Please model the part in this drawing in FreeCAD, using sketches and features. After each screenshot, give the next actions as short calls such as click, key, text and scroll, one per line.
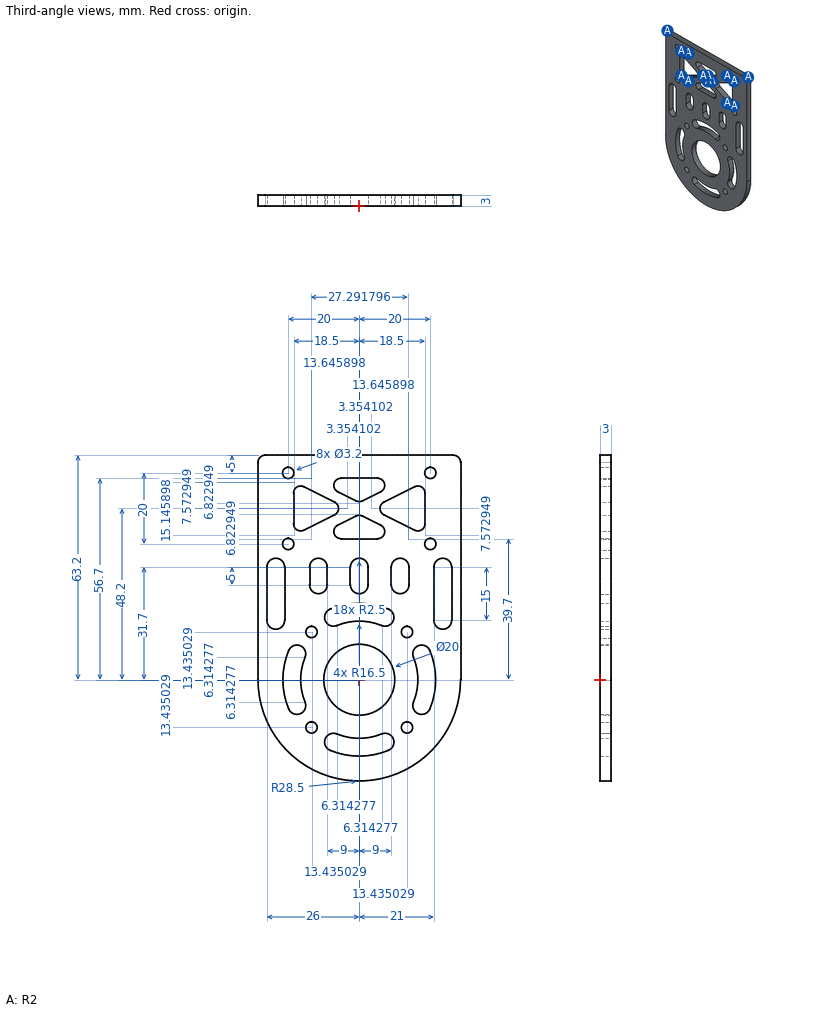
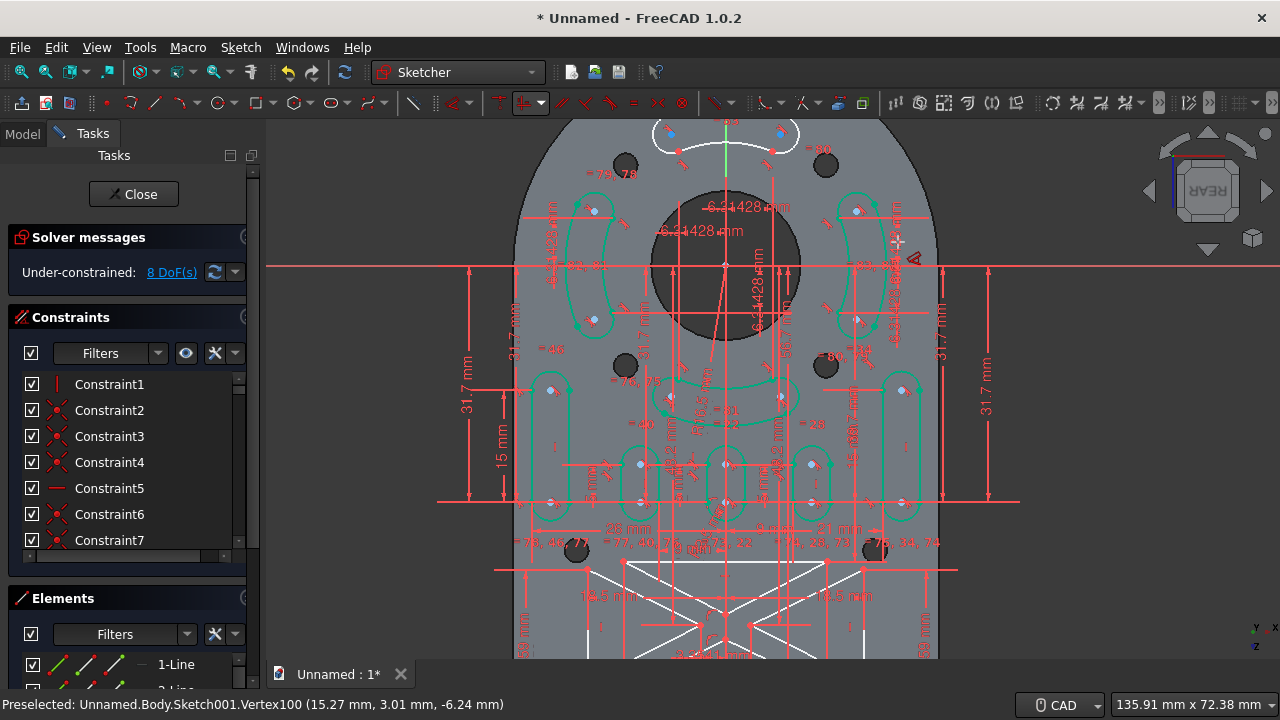
click(773, 152)
click(749, 372)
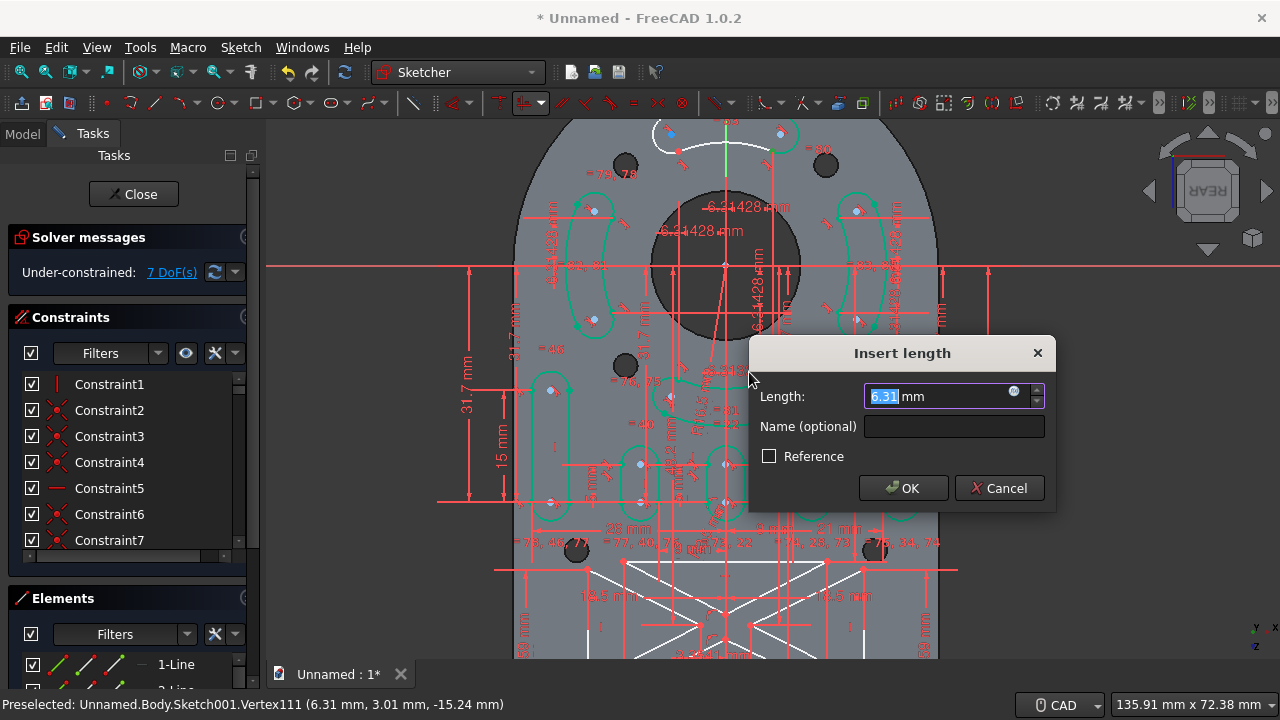
text(6.314277)
key(Return)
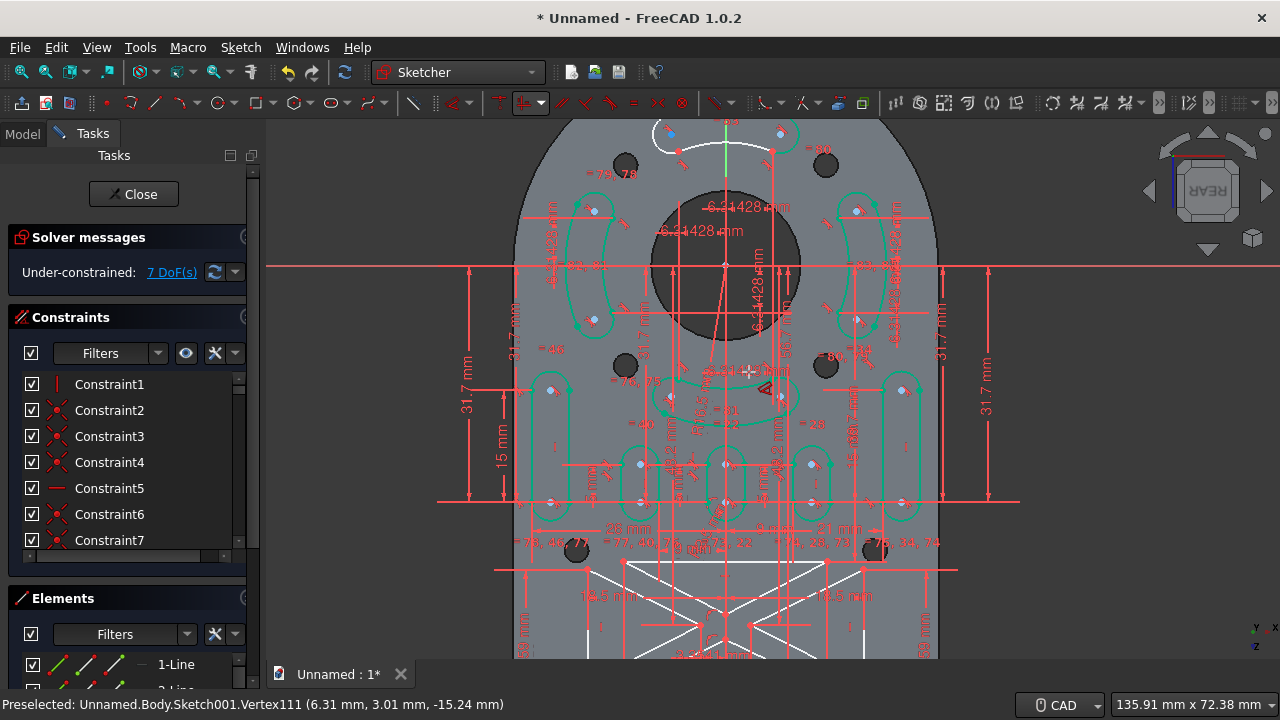
click(679, 152)
click(686, 300)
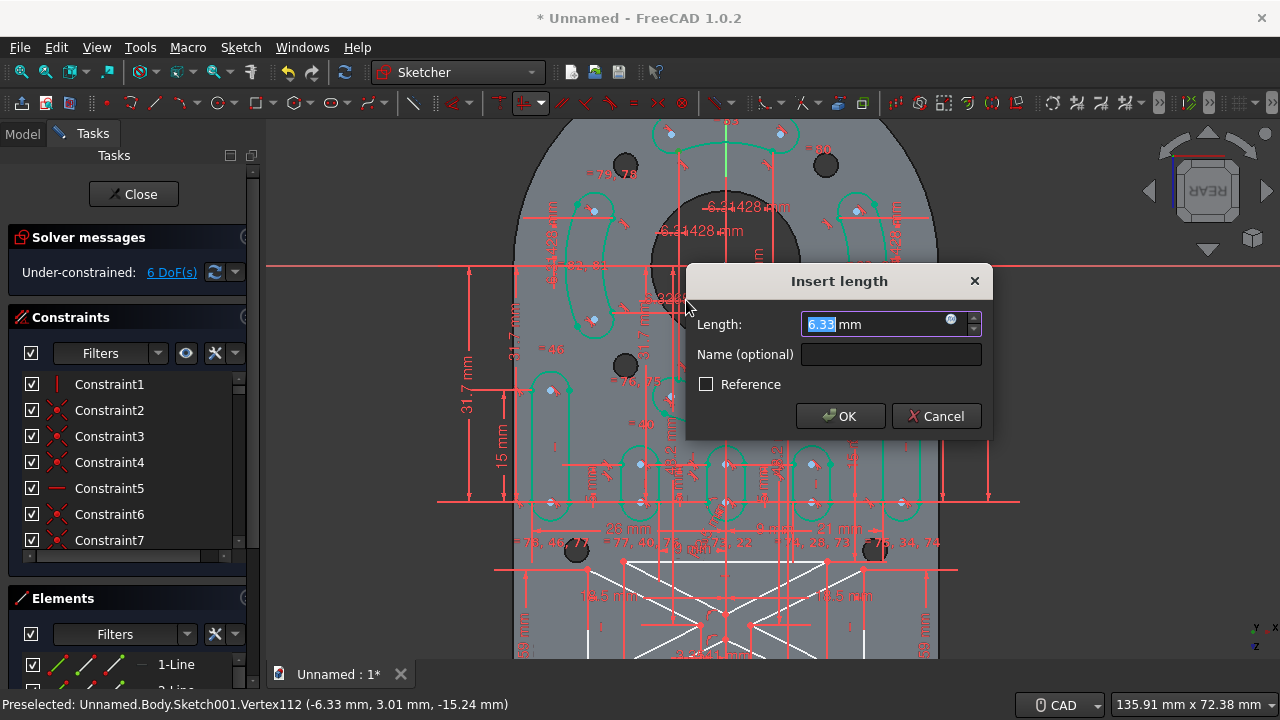
text(6.314277)
key(Return)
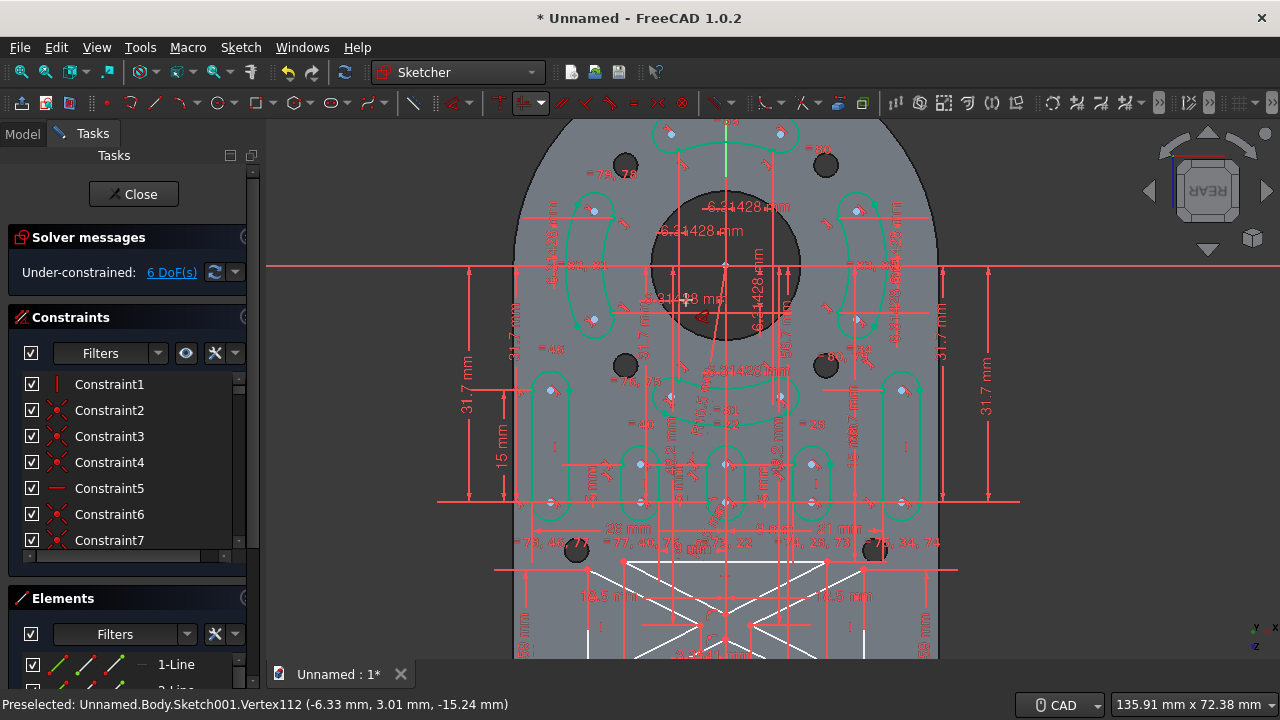
scroll(678, 379, down, 3)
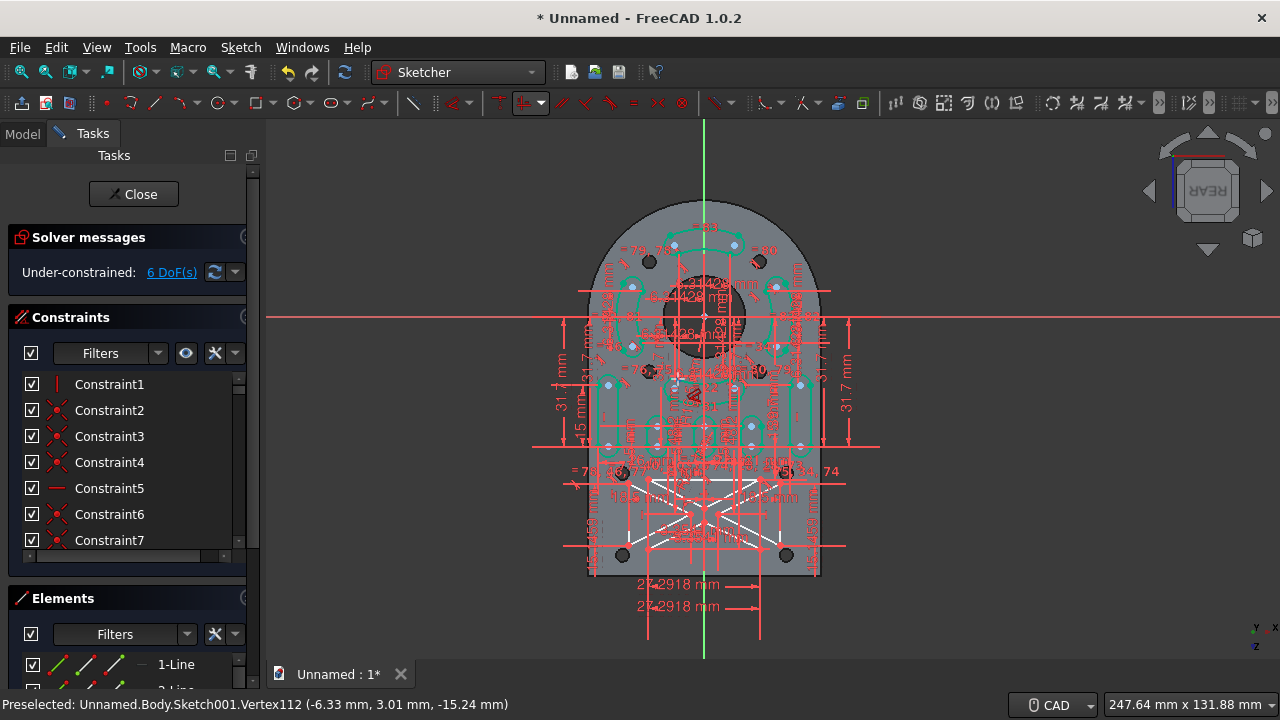
scroll(647, 536, up, 2)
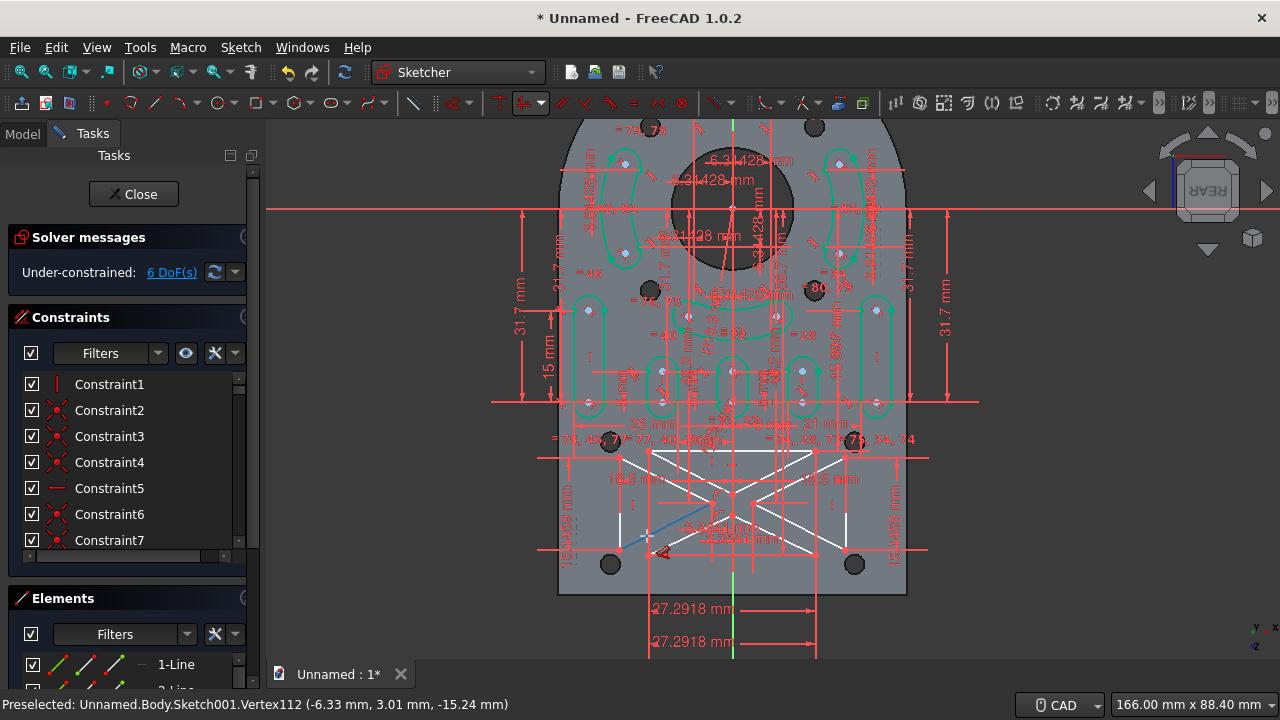
click(647, 536)
click(818, 516)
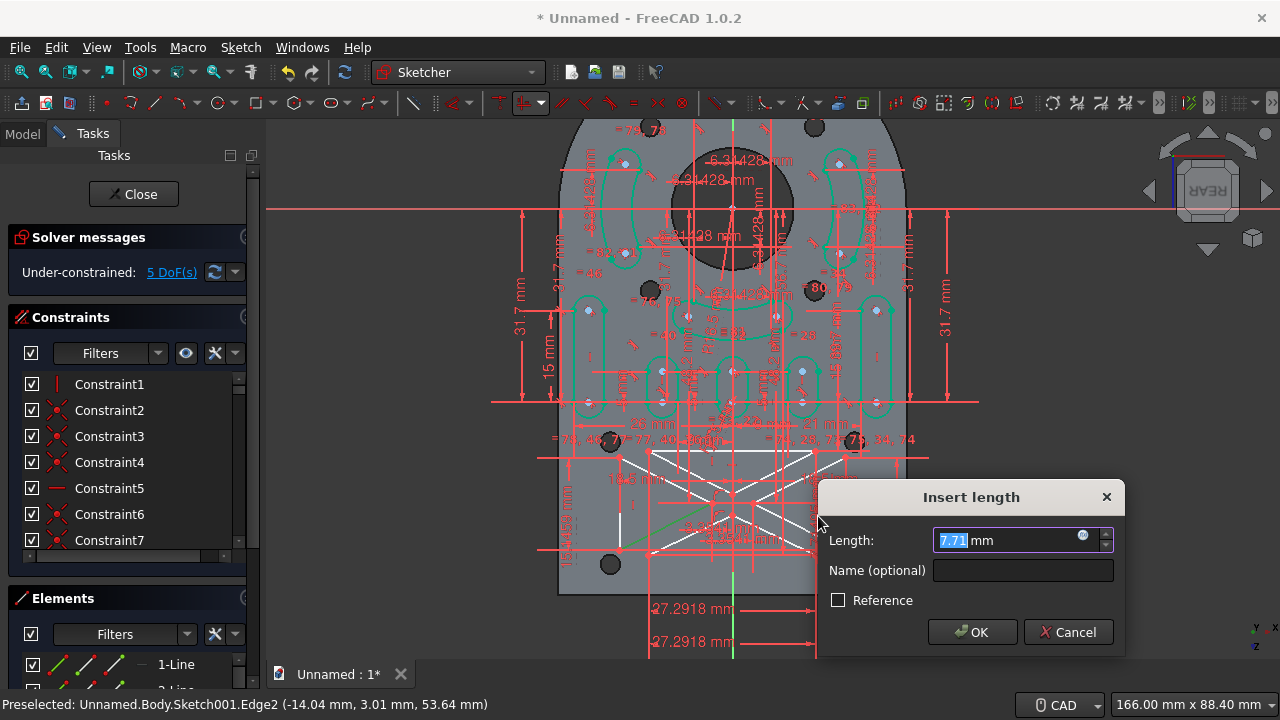
text(7.572949)
key(Return)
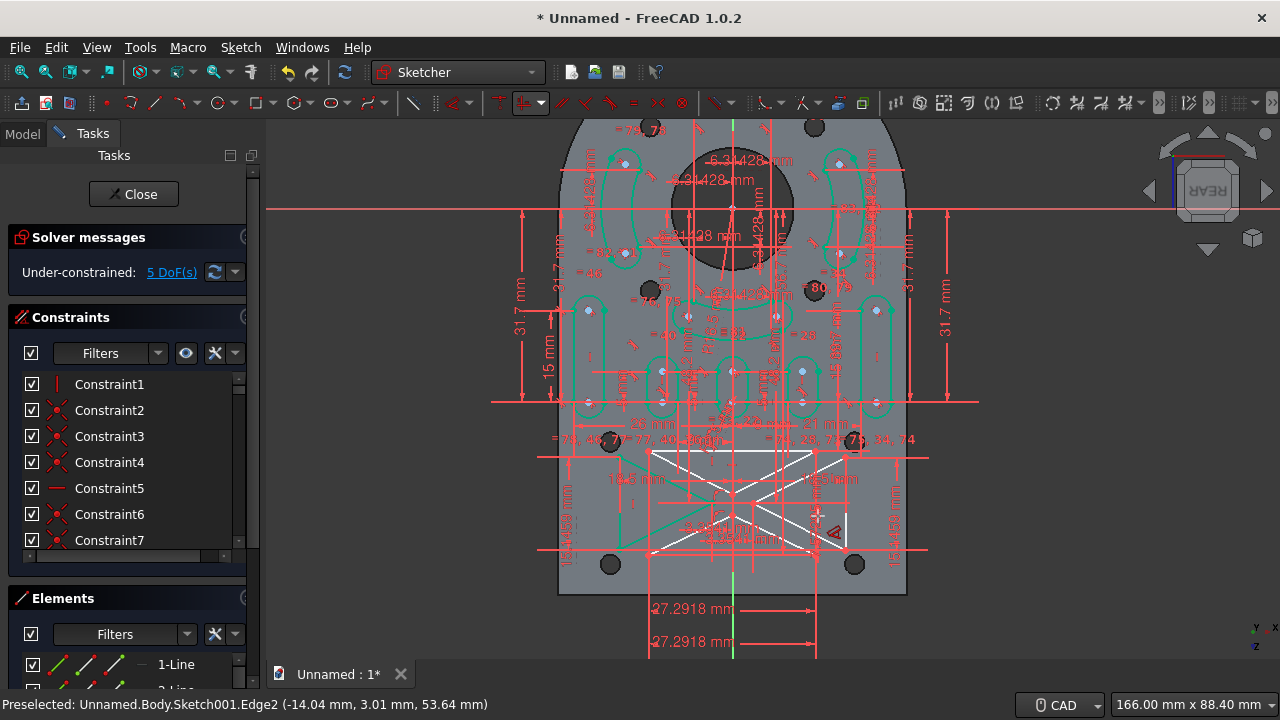
click(674, 464)
click(591, 458)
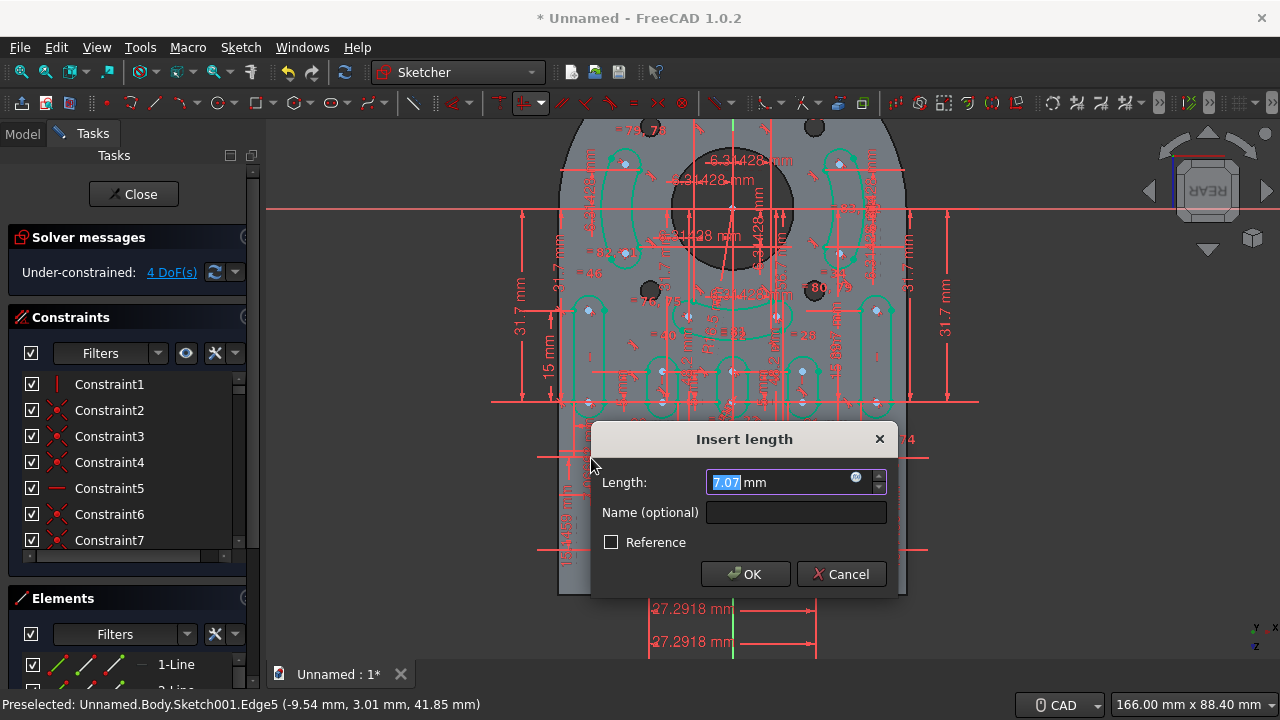
text(6.822949)
key(Return)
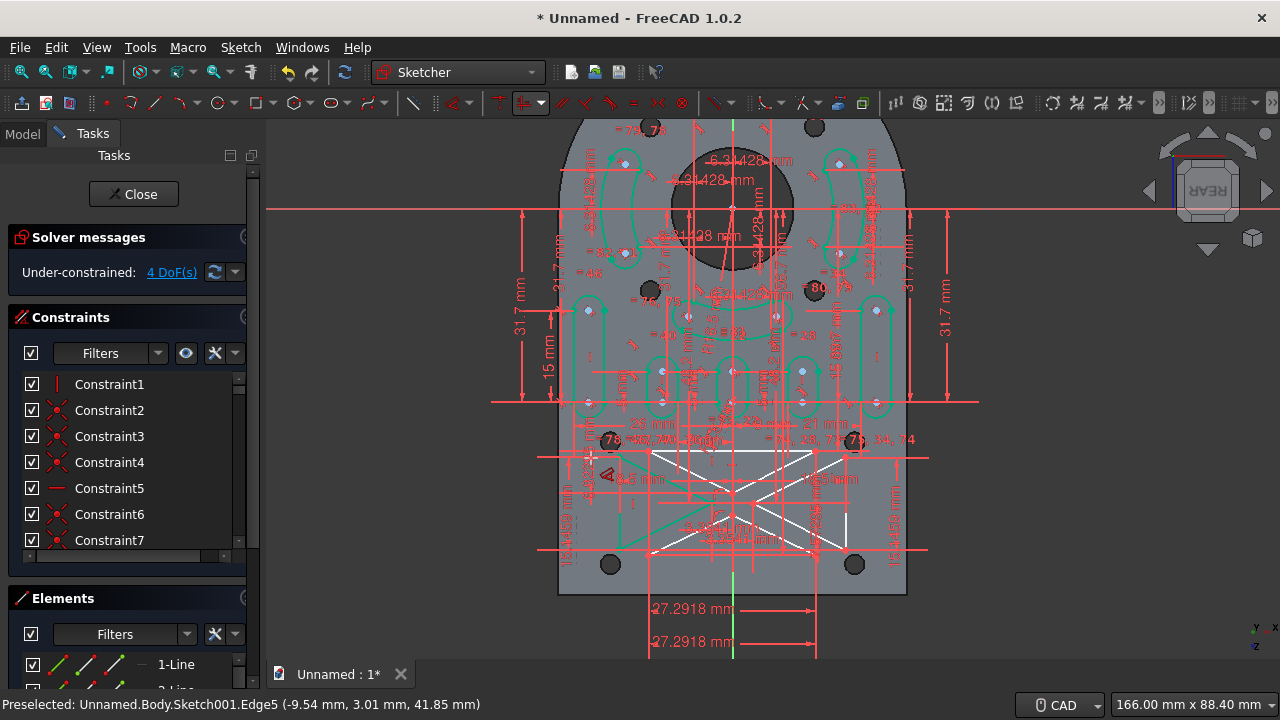
click(818, 472)
click(719, 470)